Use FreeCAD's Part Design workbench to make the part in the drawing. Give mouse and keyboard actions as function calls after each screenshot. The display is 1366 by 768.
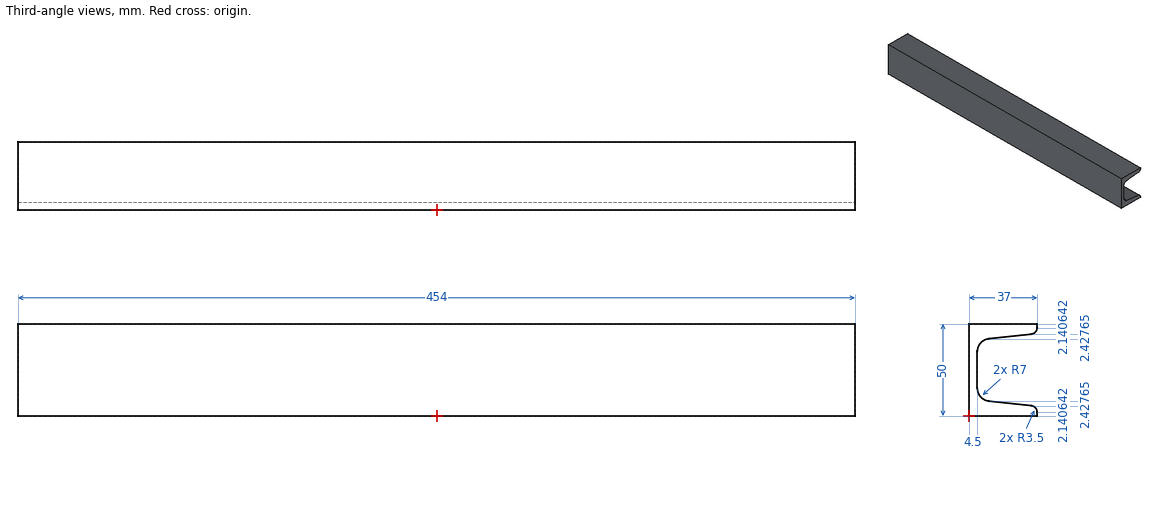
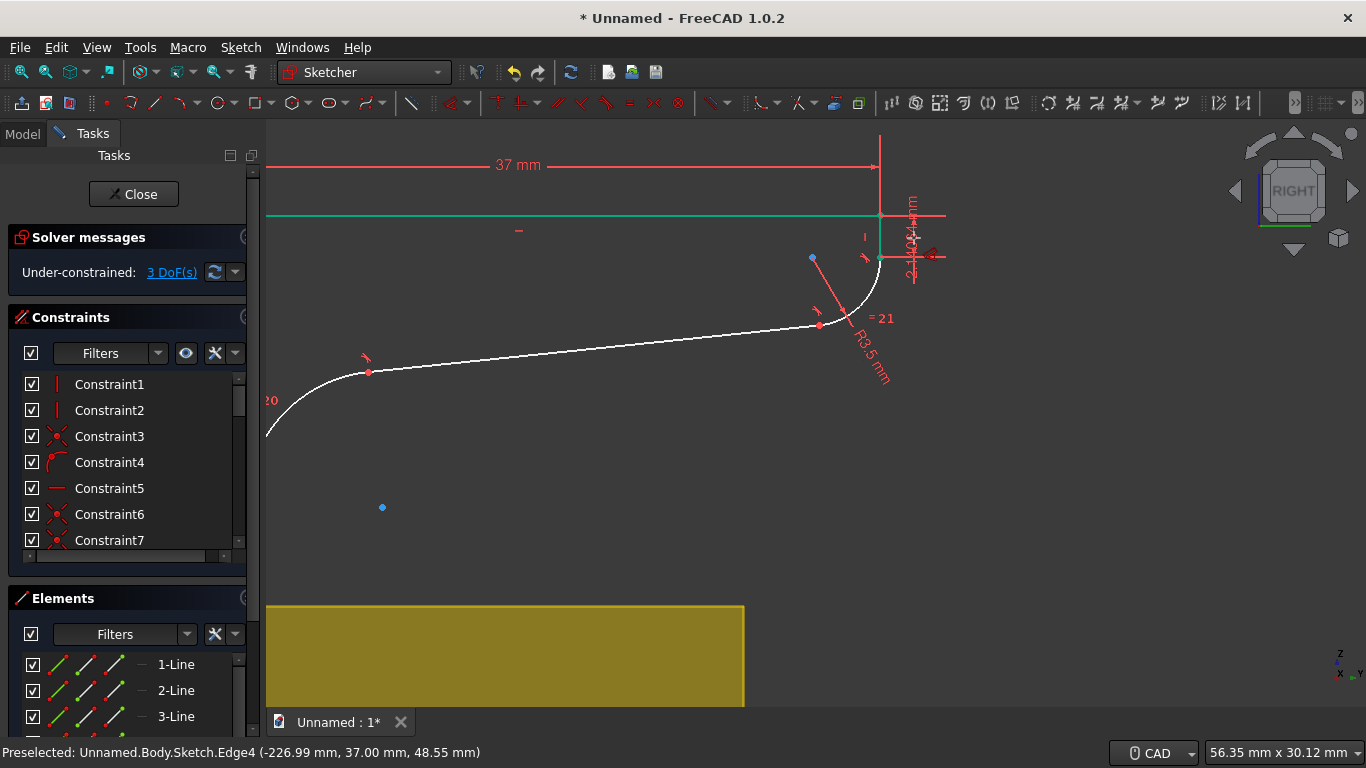
scroll(880, 244, down, 5)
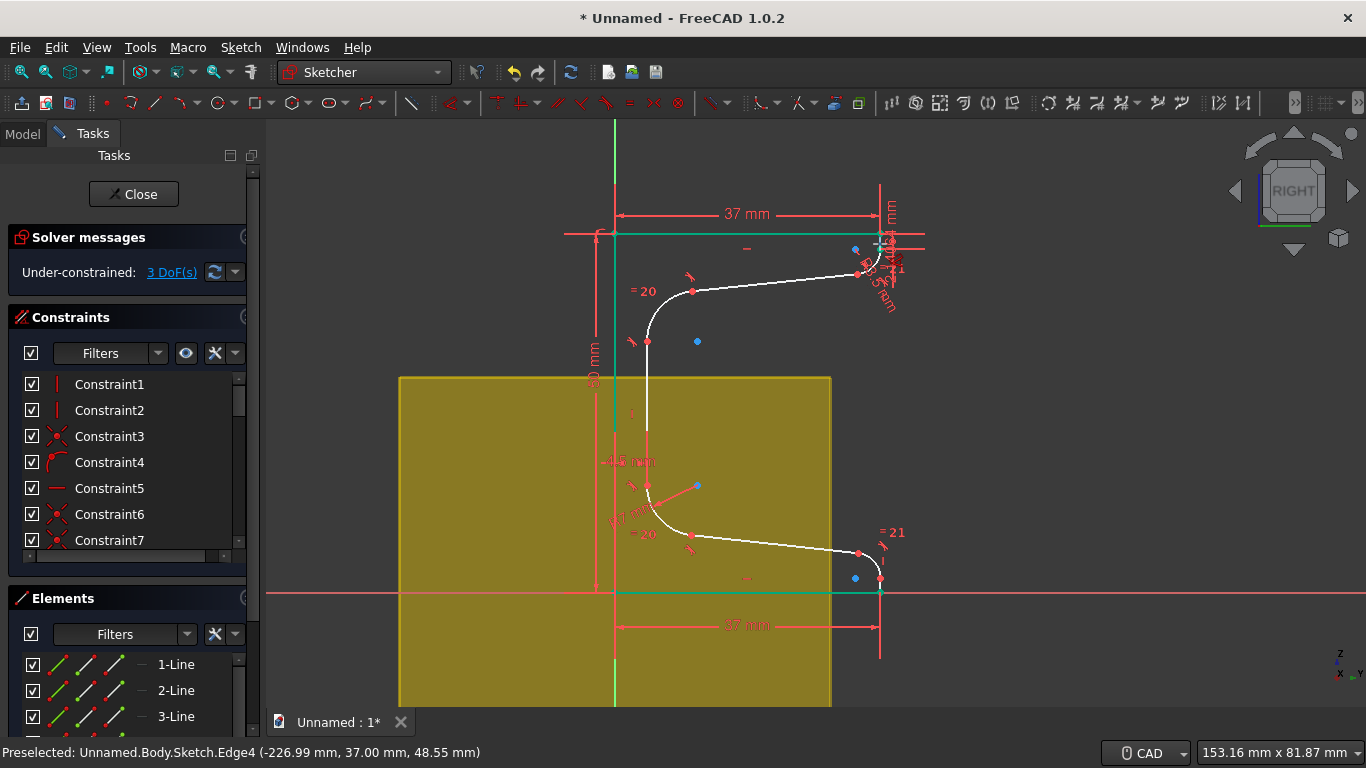
scroll(880, 588, up, 6)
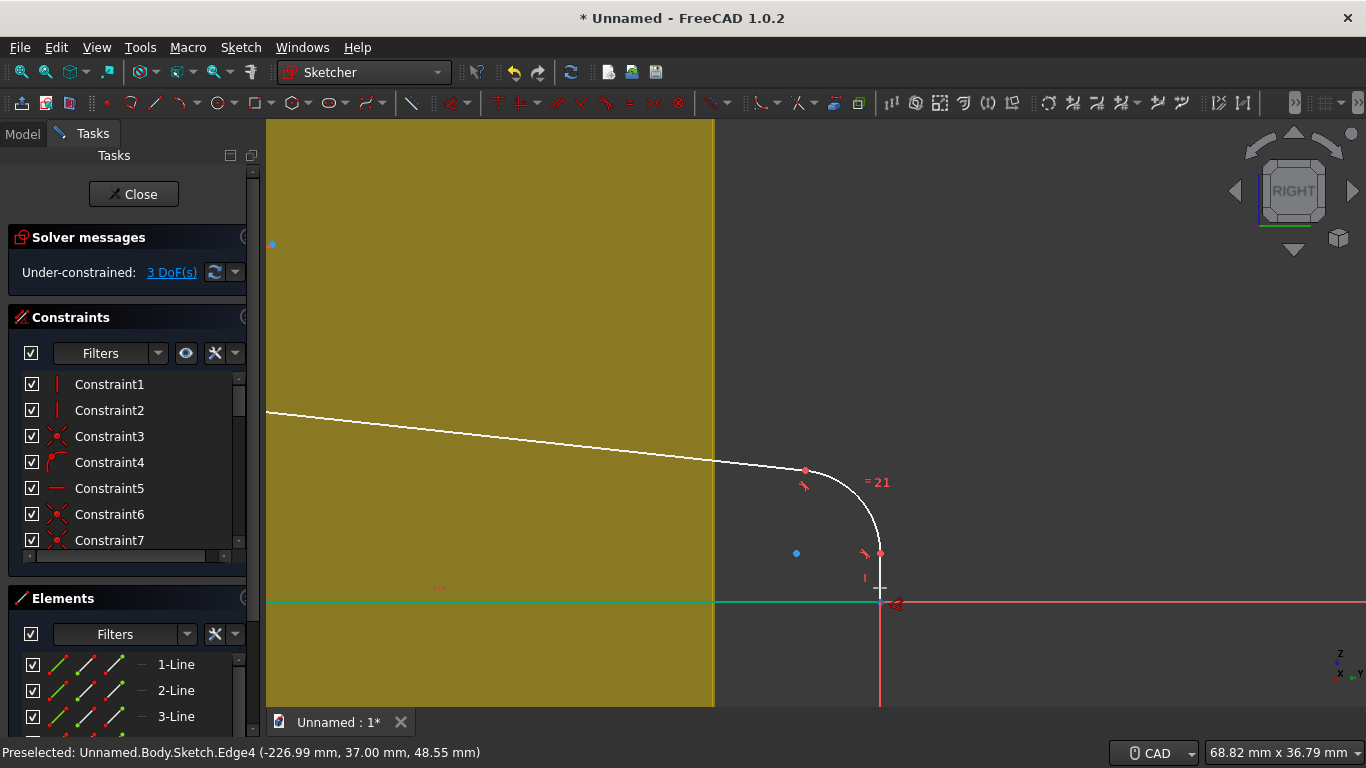
click(880, 588)
click(914, 578)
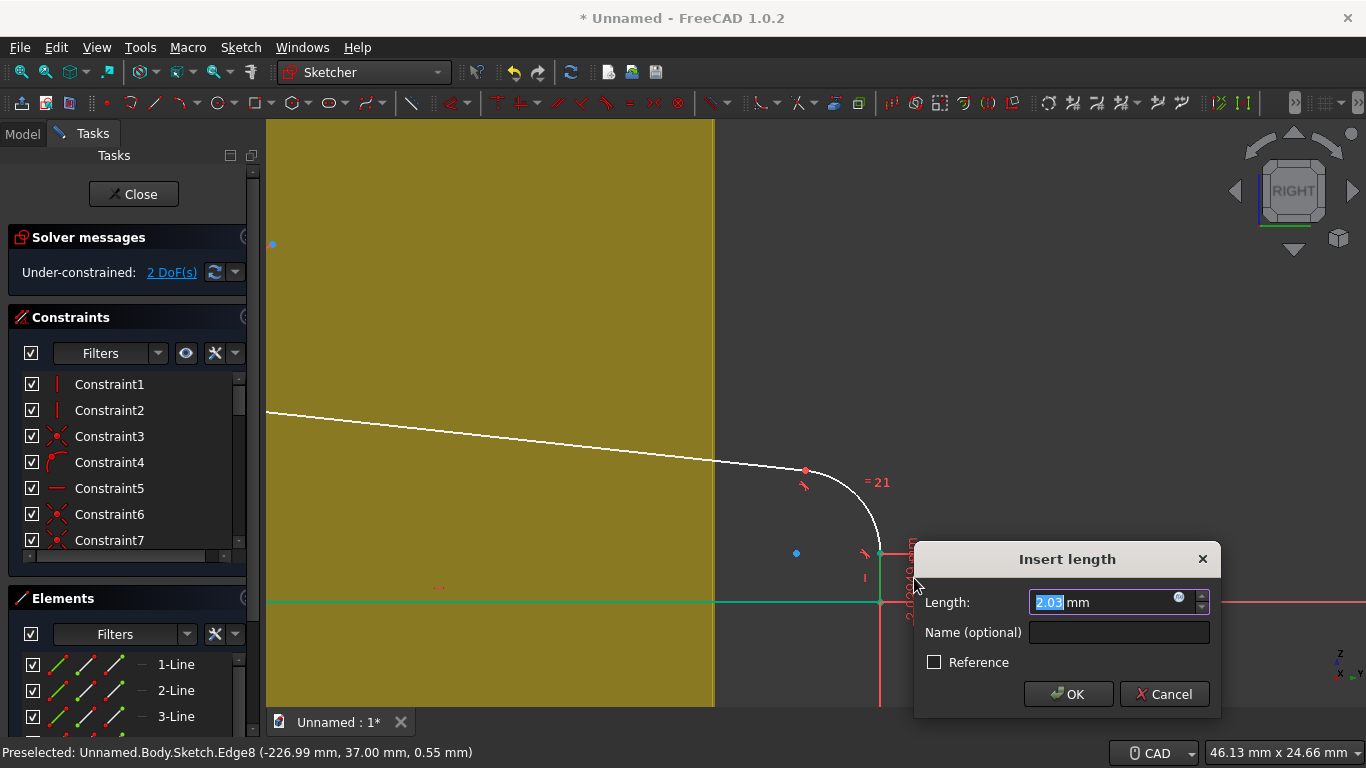
text(2.140642)
key(Return)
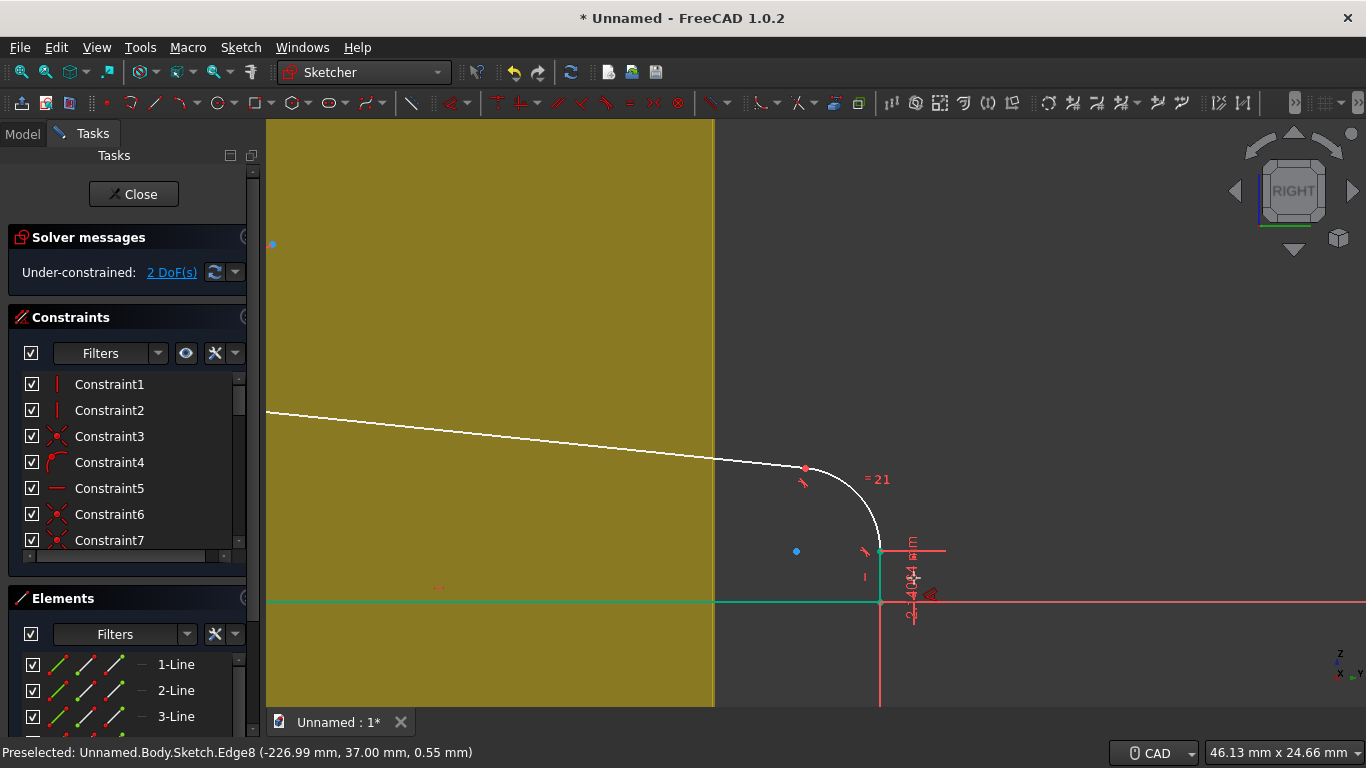
click(640, 451)
click(839, 440)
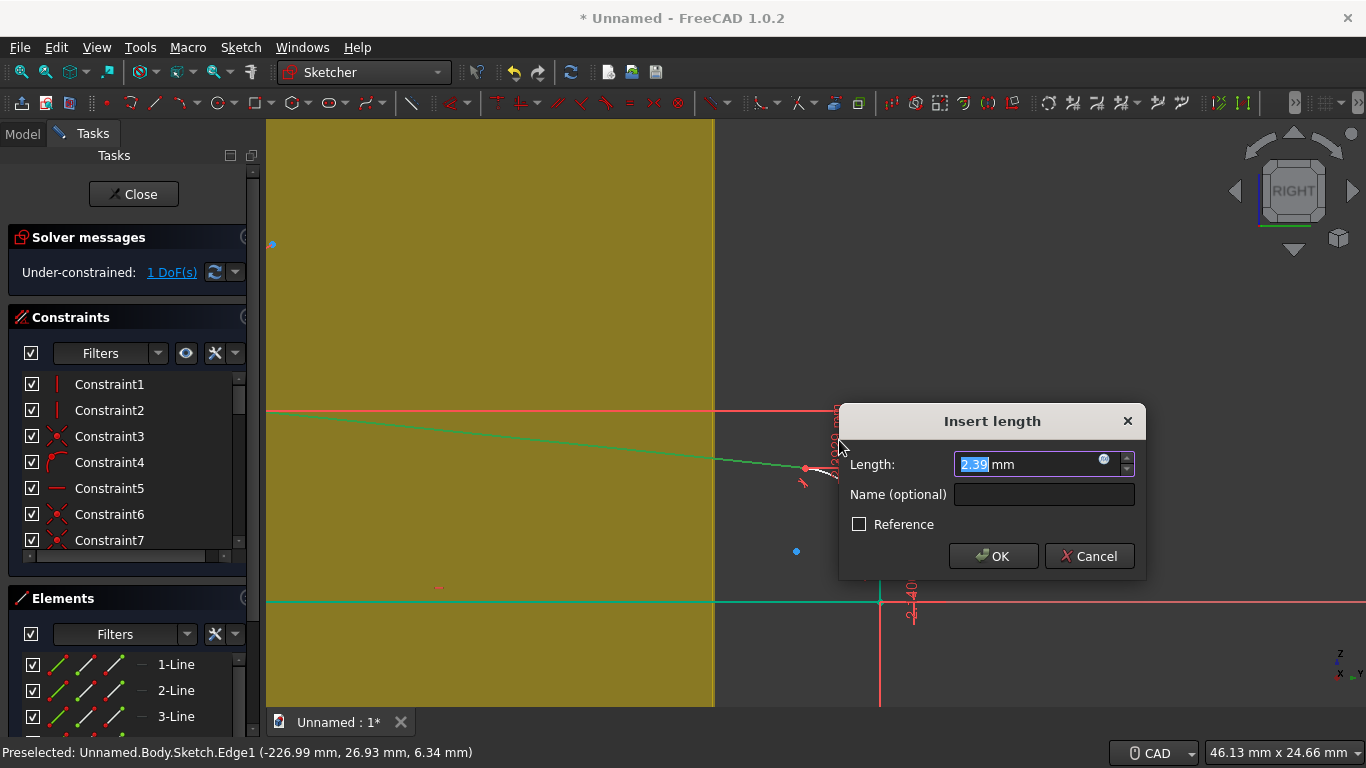
text(2.42765)
key(Return)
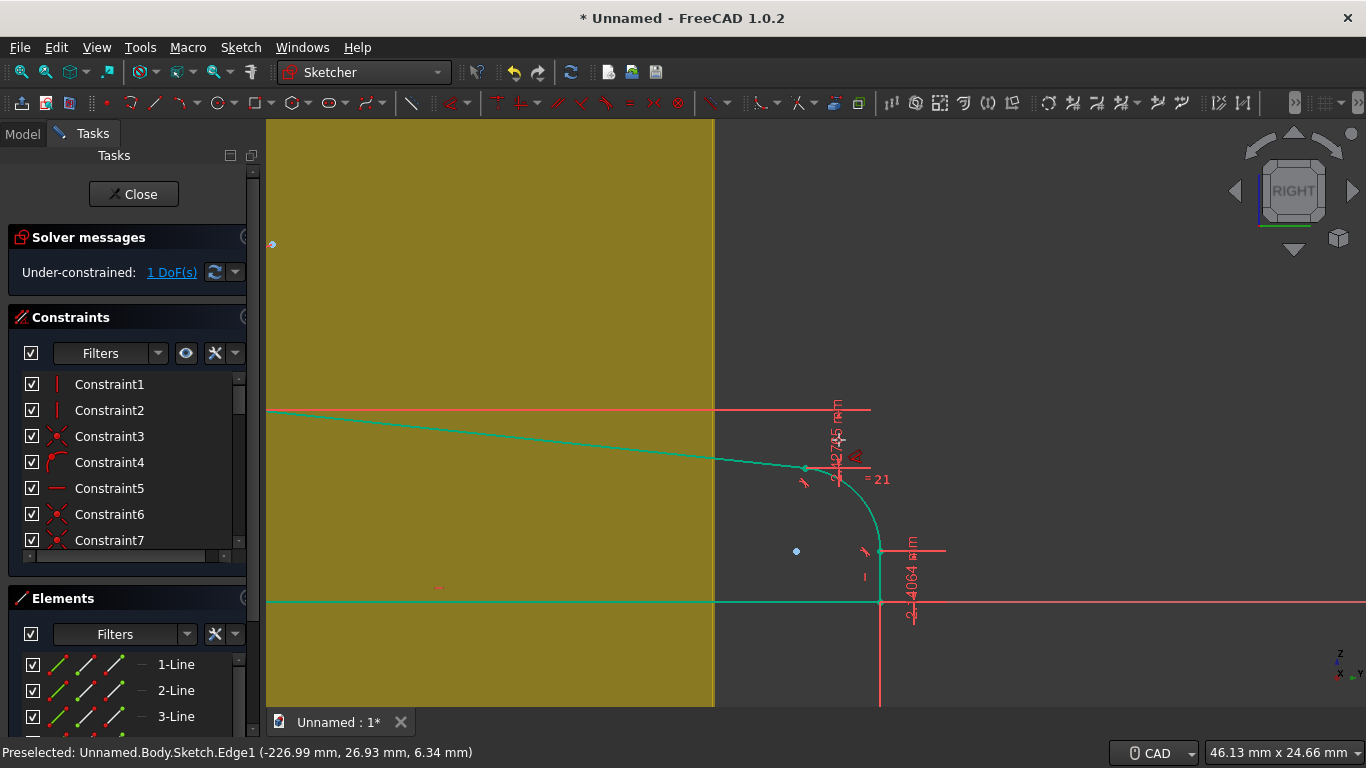
scroll(880, 588, down, 6)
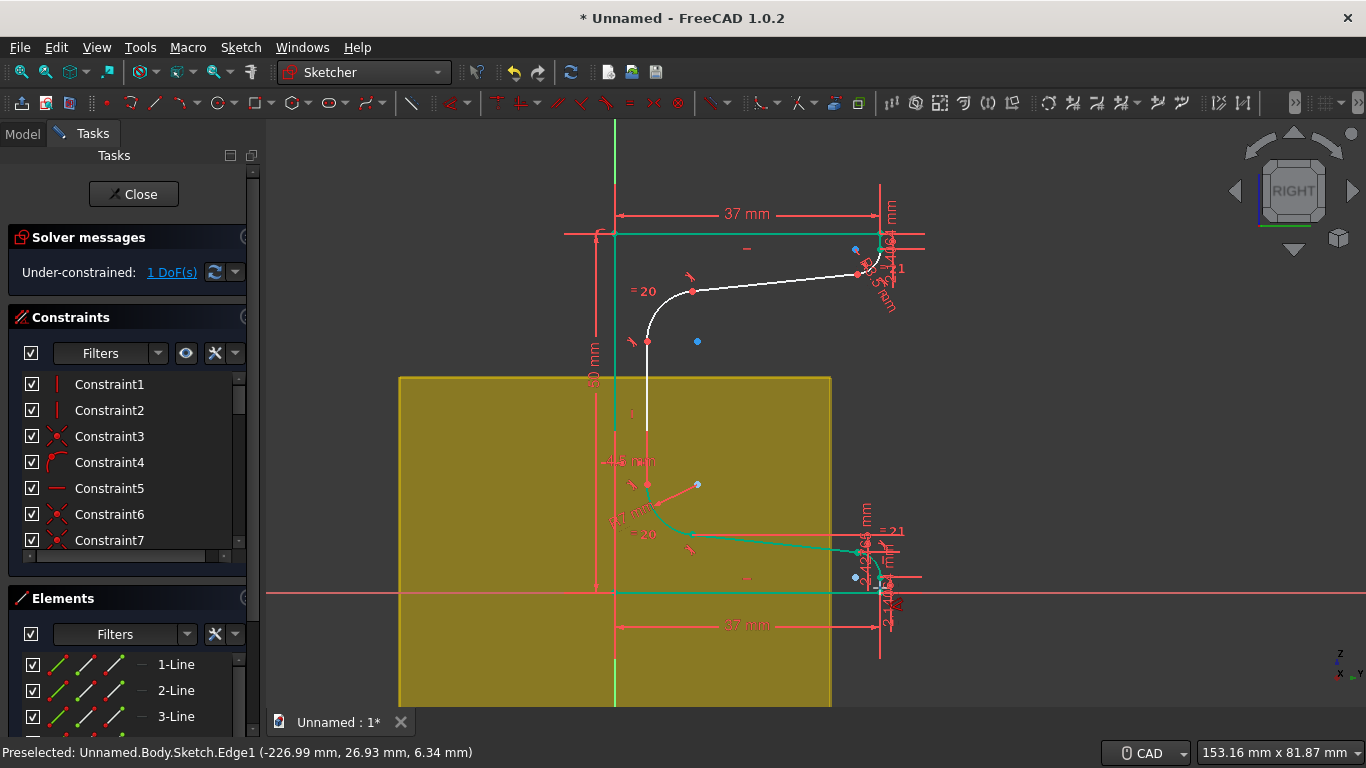
scroll(742, 286, up, 5)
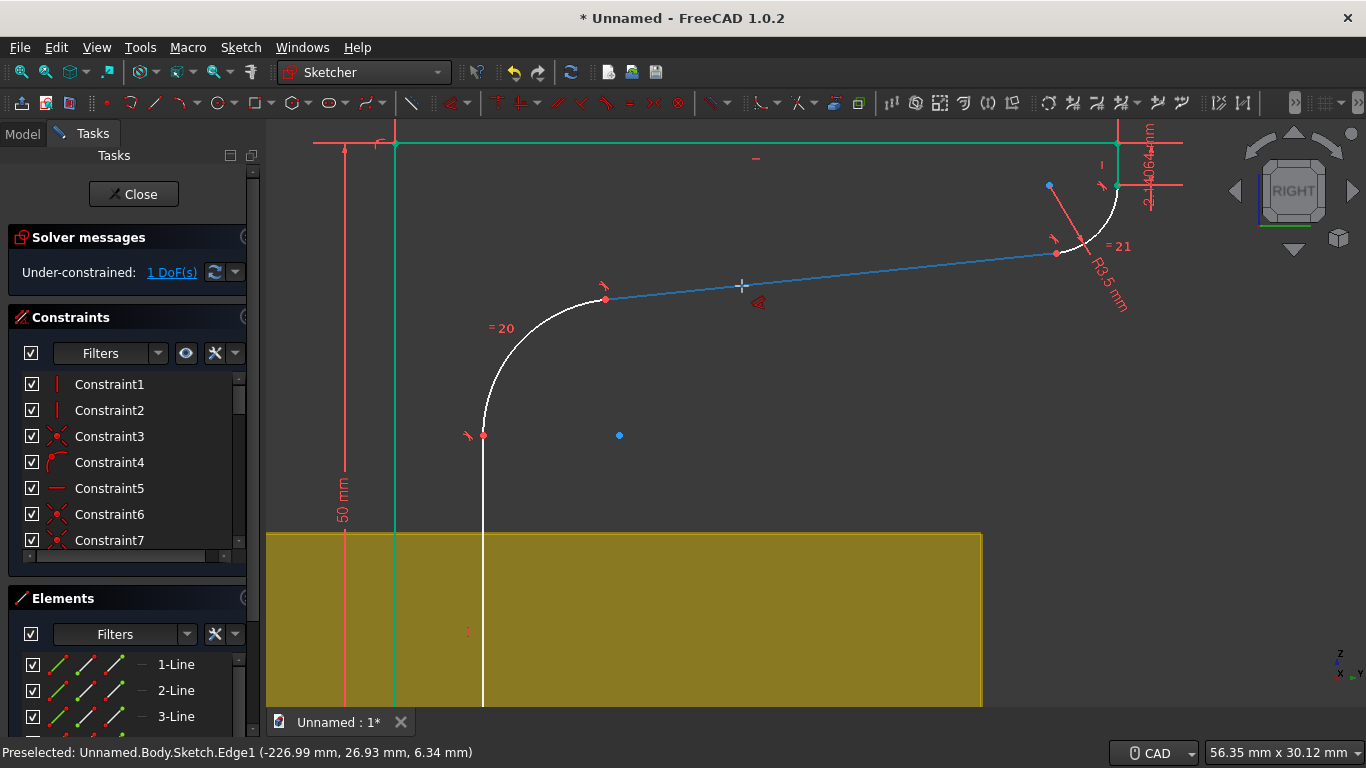
click(741, 286)
click(1090, 266)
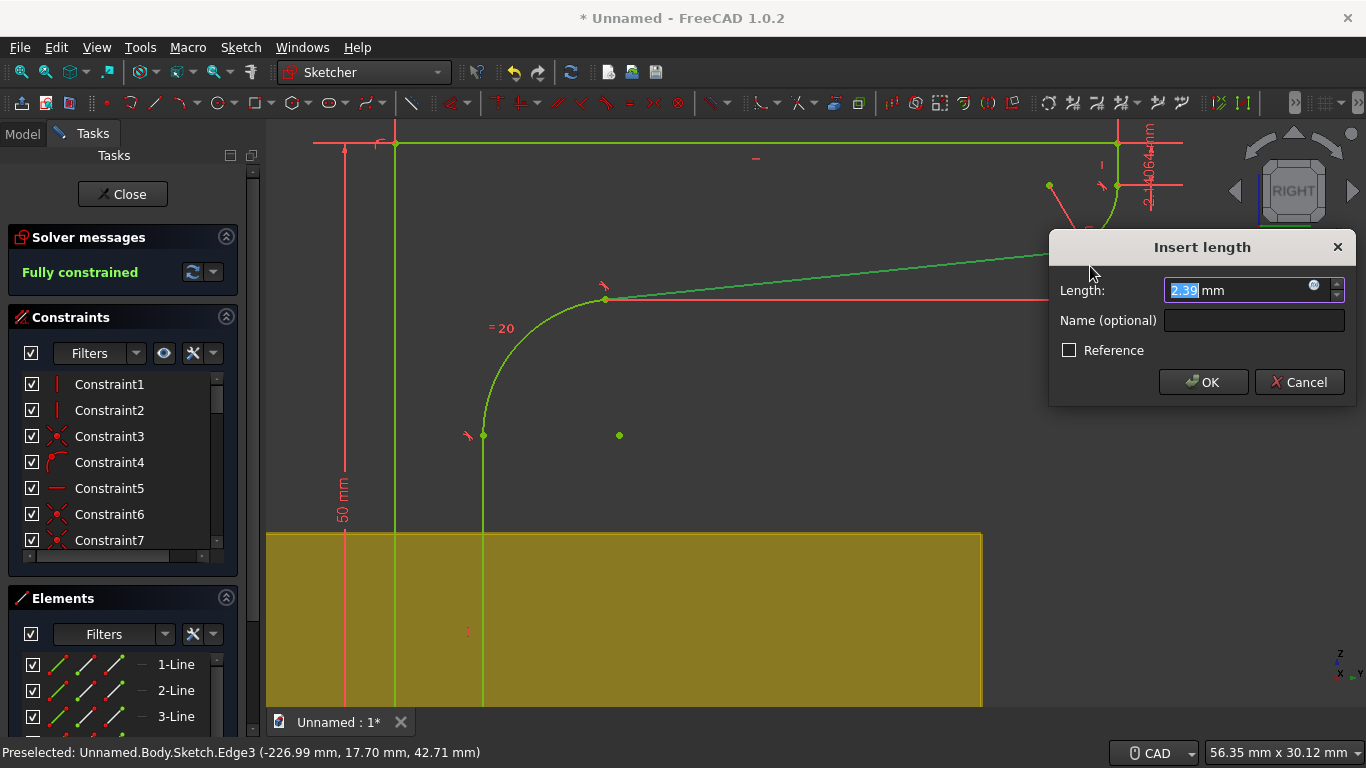
text(2.42765)
key(Return)
key(Escape)